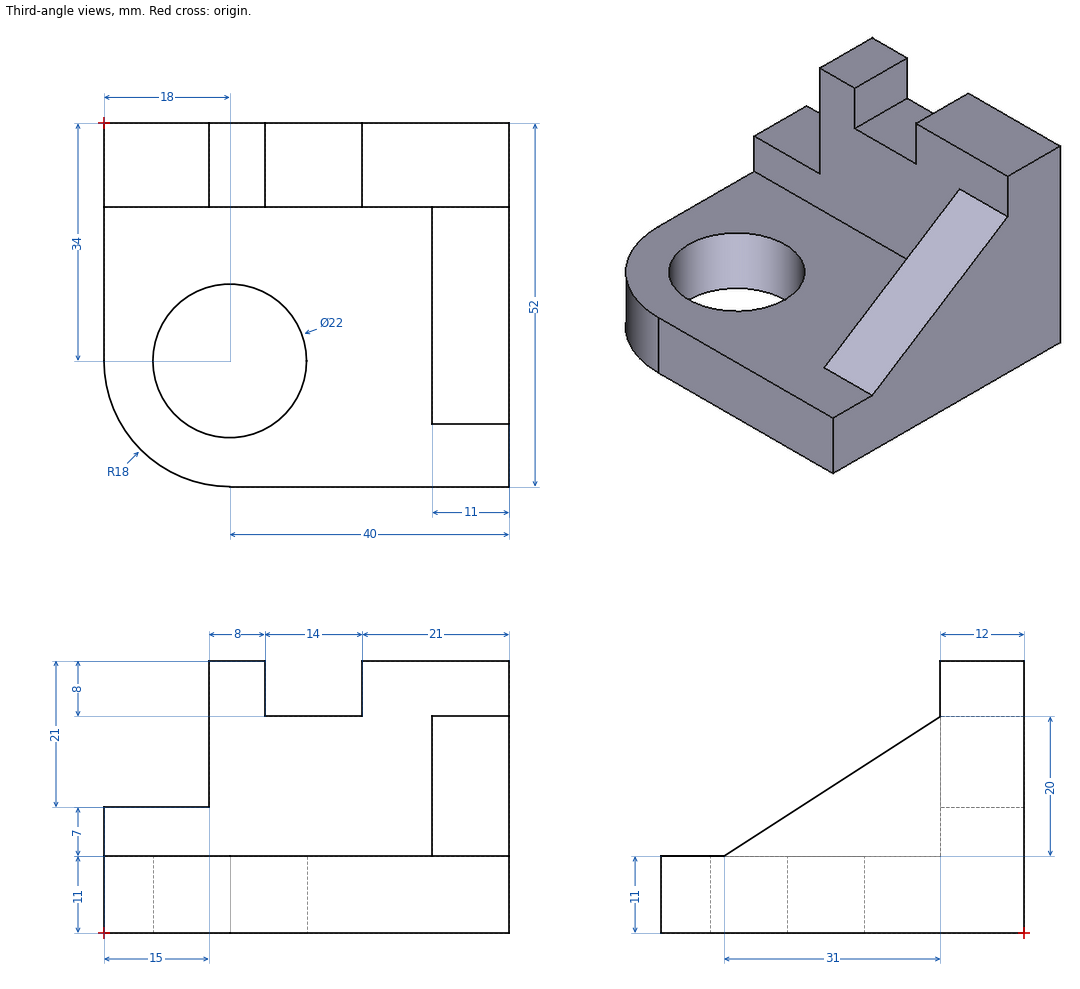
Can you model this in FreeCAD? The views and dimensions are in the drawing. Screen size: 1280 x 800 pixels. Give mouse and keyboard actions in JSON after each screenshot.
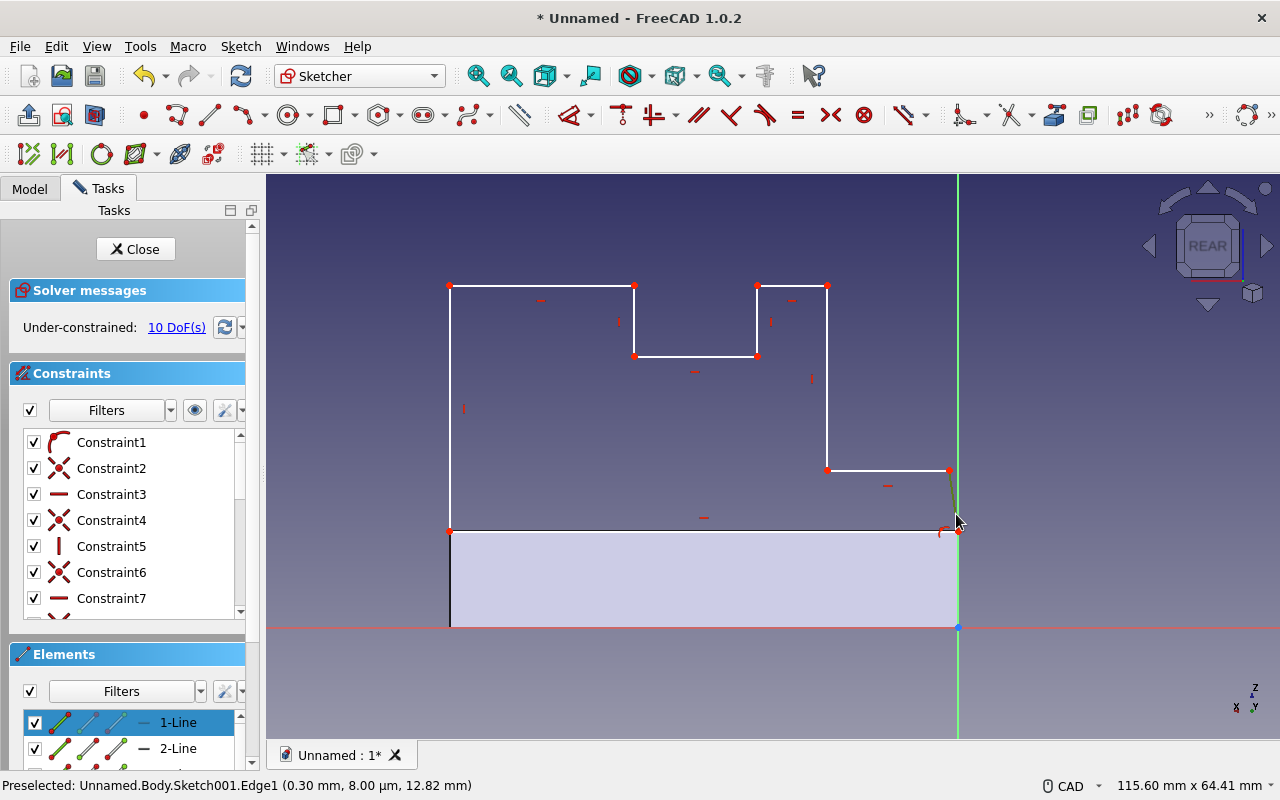
{"action": "left_click", "coordinate": [676, 116]}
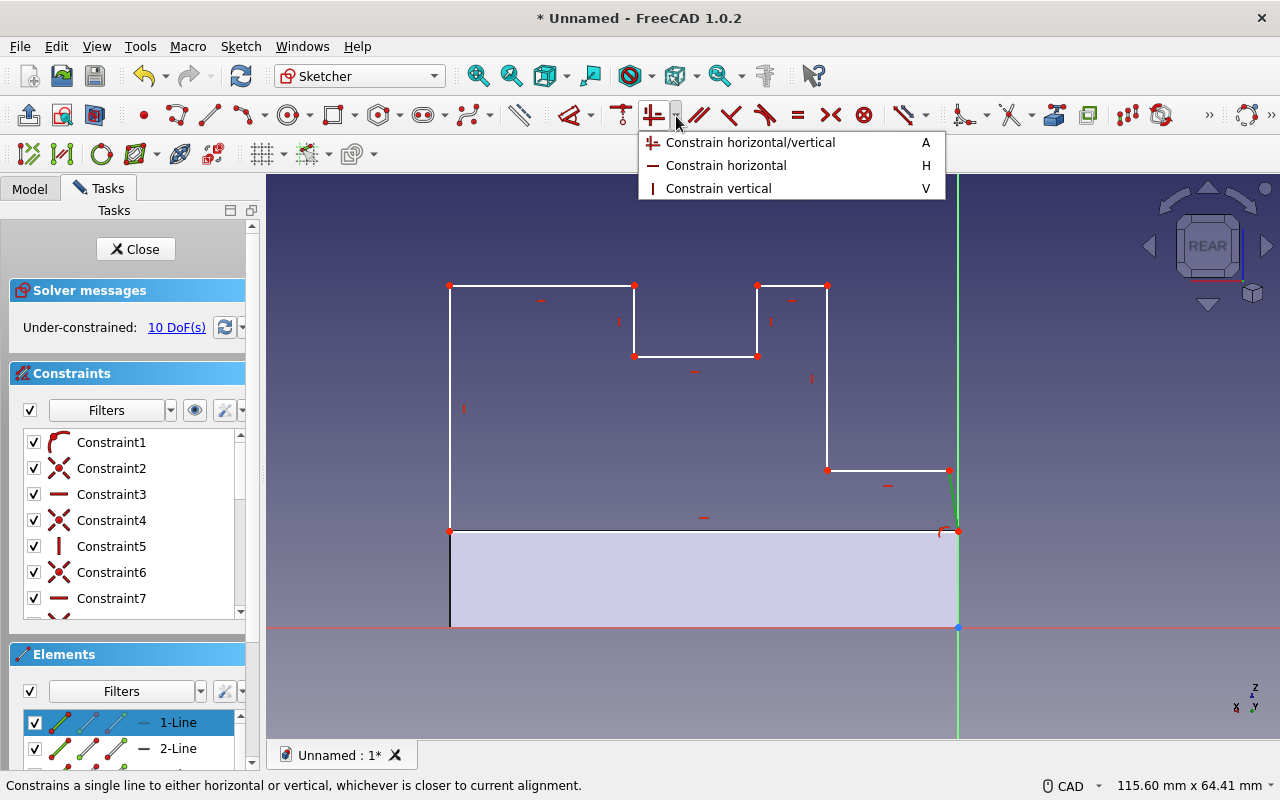
{"action": "left_click", "coordinate": [792, 188]}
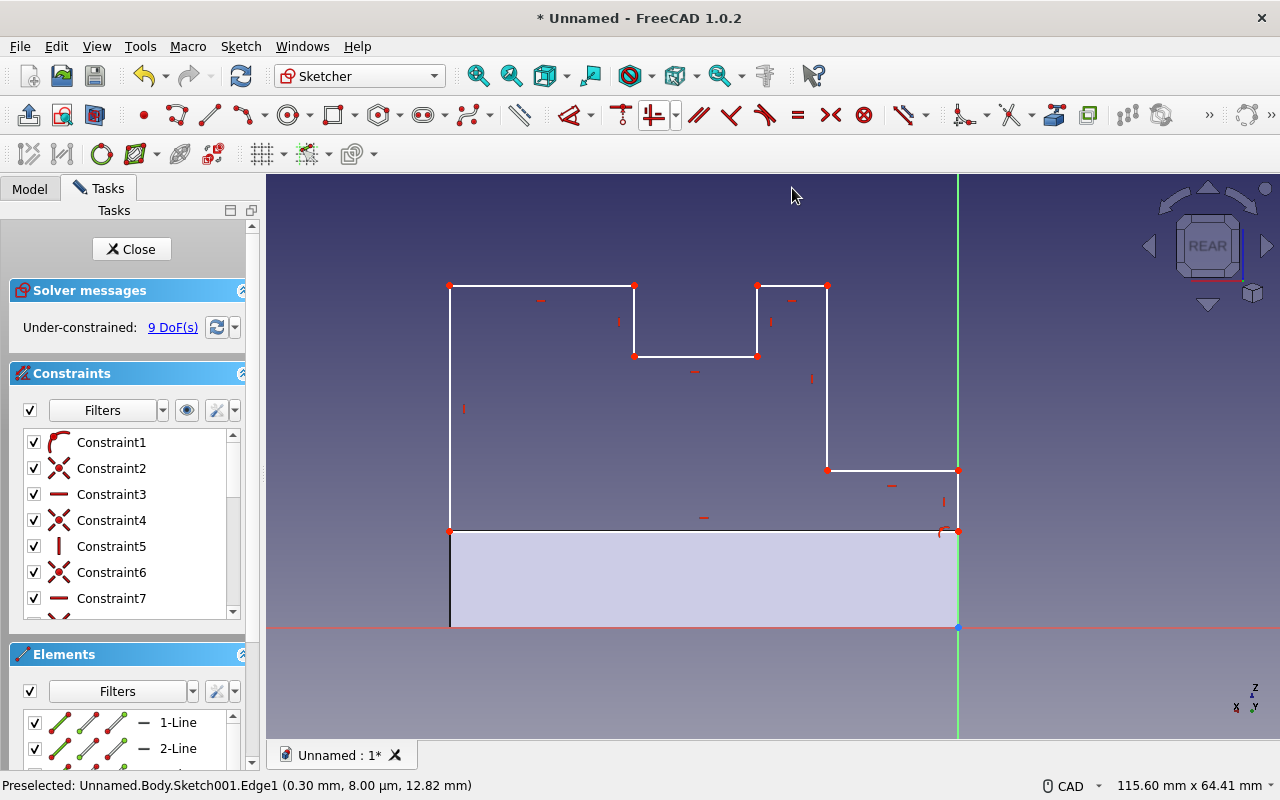
{"action": "left_click", "coordinate": [568, 116]}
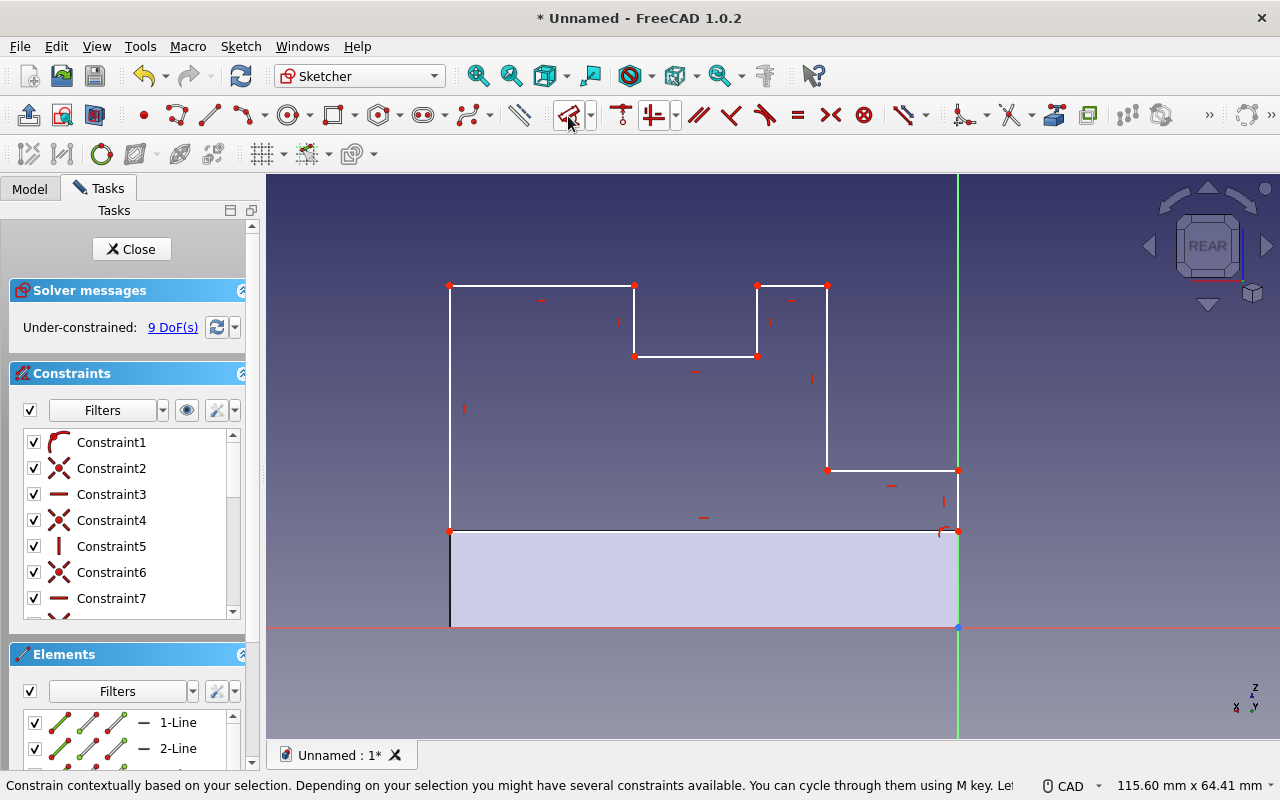
{"action": "left_click", "coordinate": [958, 514]}
{"action": "left_click", "coordinate": [992, 501]}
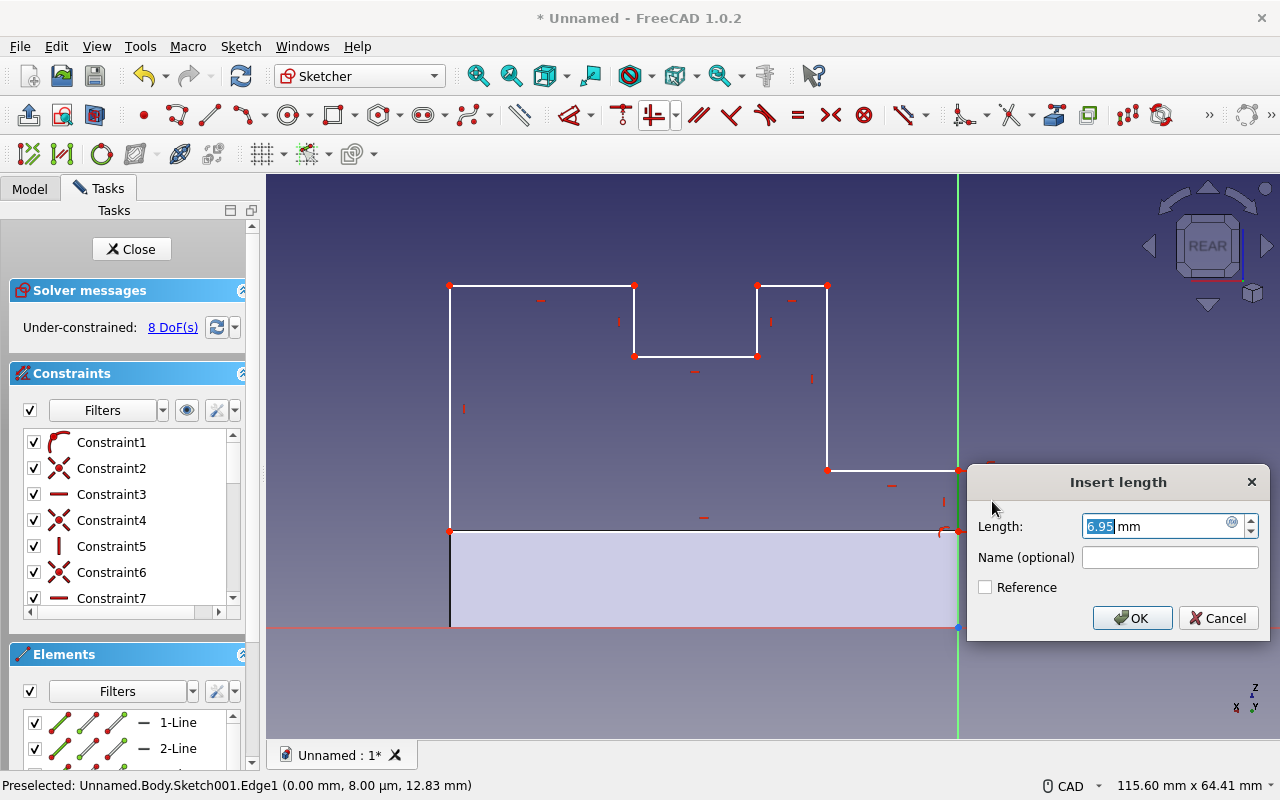
{"action": "type", "text": "7"}
{"action": "key", "text": "Return"}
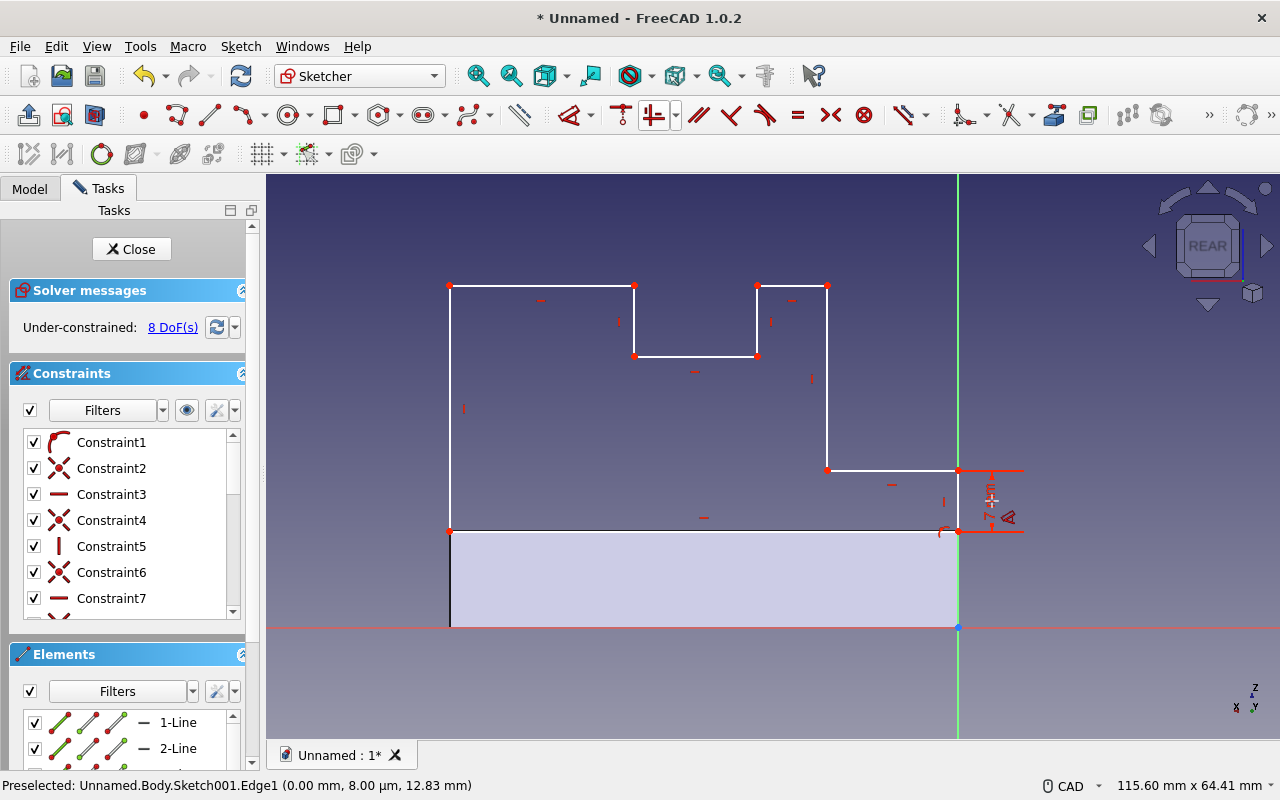
{"action": "left_click", "coordinate": [806, 286]}
{"action": "left_click", "coordinate": [792, 252]}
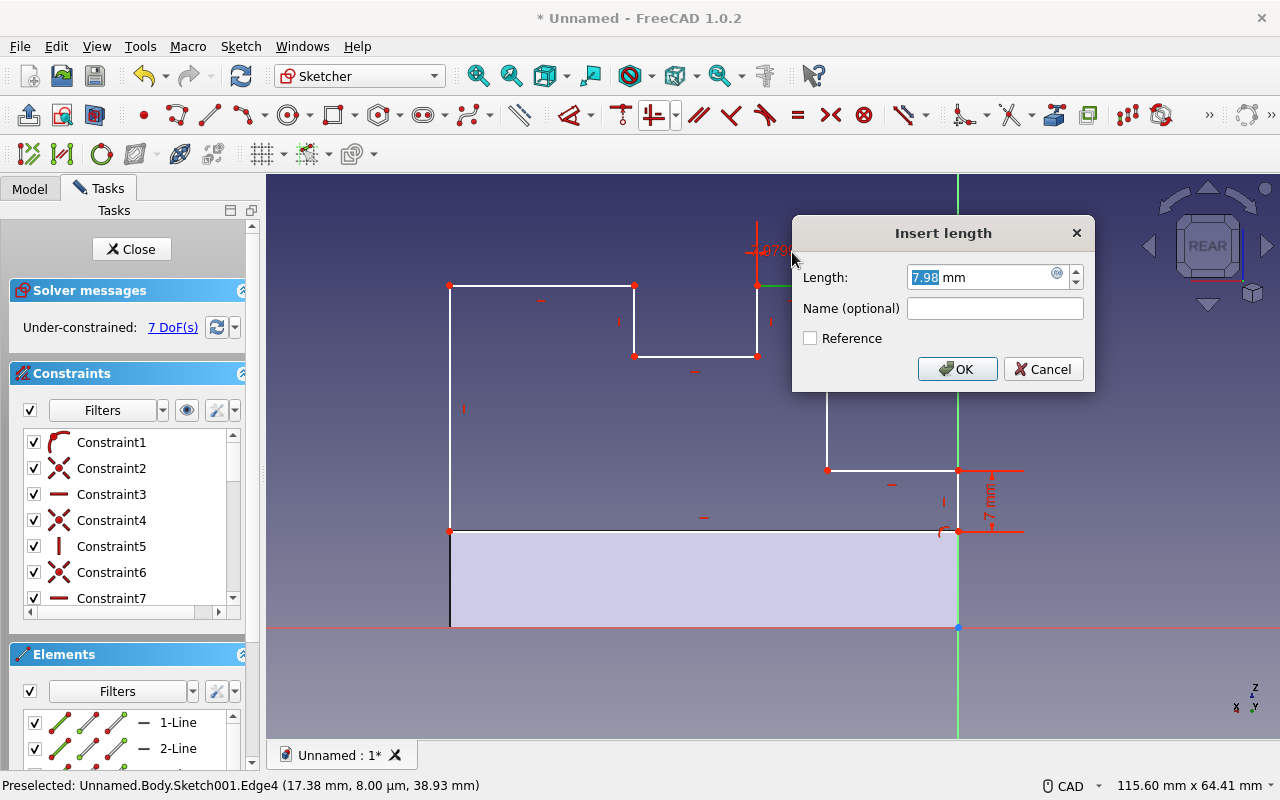
{"action": "type", "text": "8"}
{"action": "key", "text": "Return"}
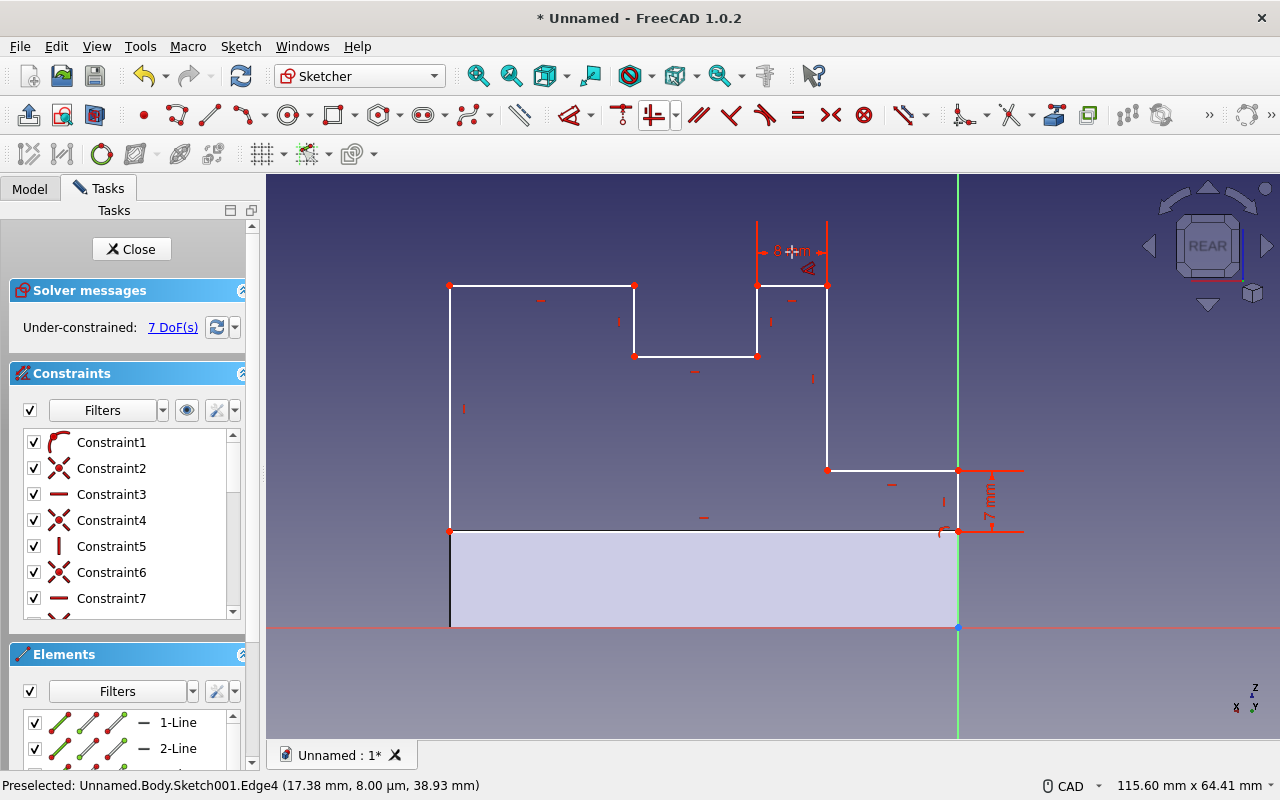
{"action": "left_click", "coordinate": [757, 307]}
{"action": "left_click", "coordinate": [791, 321]}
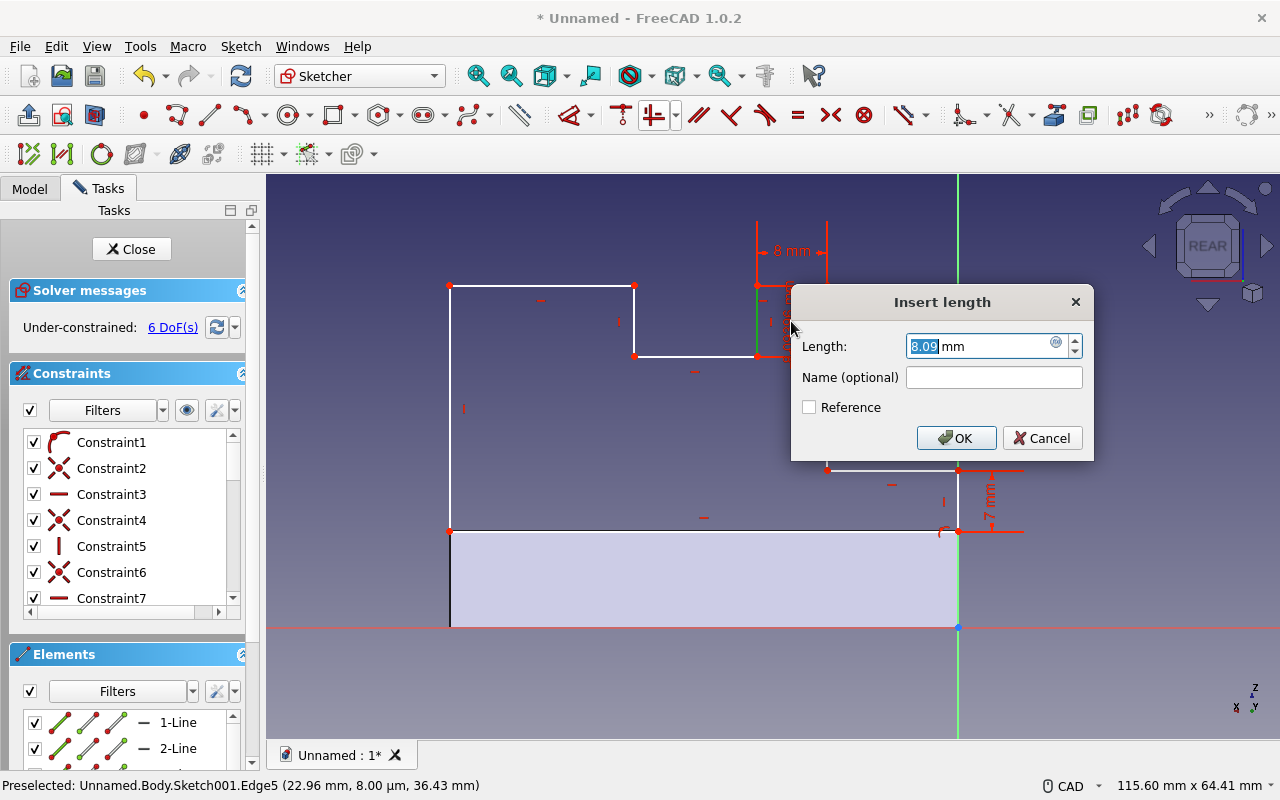
{"action": "type", "text": "8"}
{"action": "key", "text": "Return"}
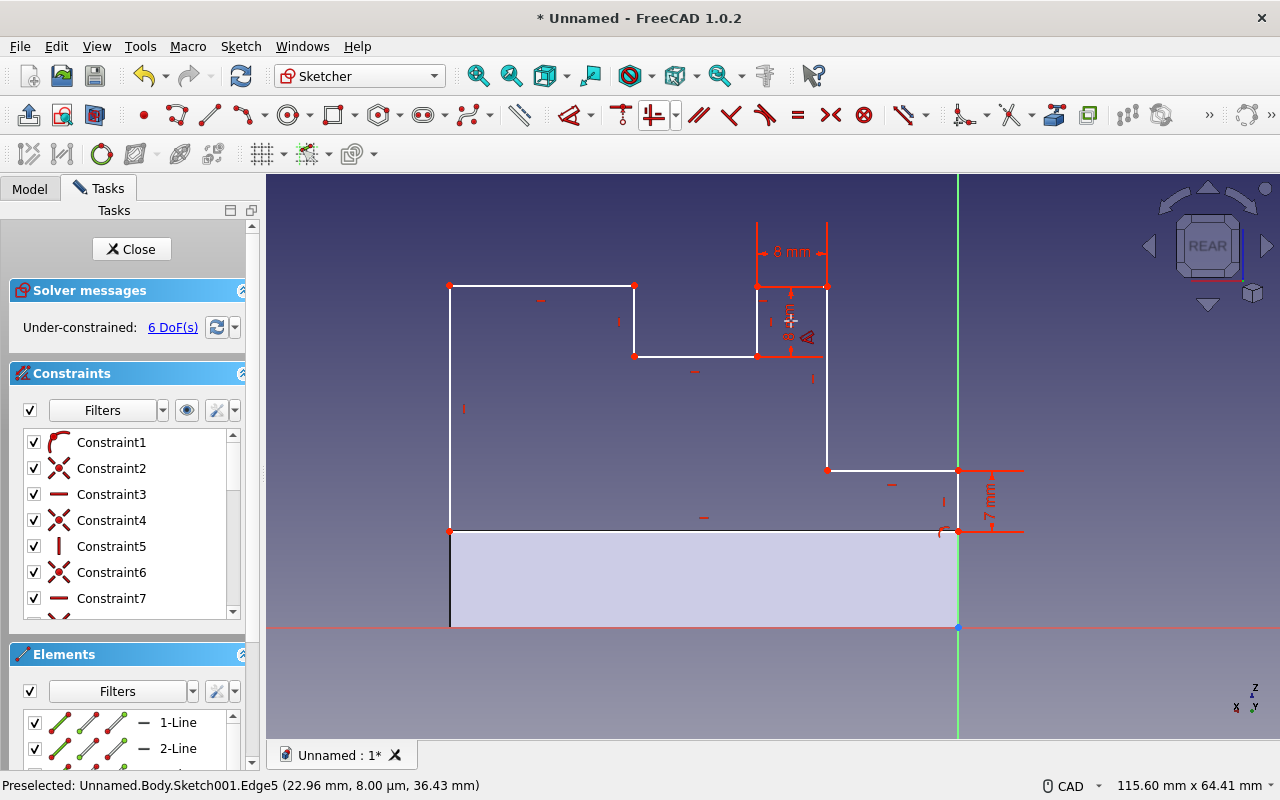
{"action": "left_click", "coordinate": [634, 336]}
{"action": "left_click", "coordinate": [600, 321]}